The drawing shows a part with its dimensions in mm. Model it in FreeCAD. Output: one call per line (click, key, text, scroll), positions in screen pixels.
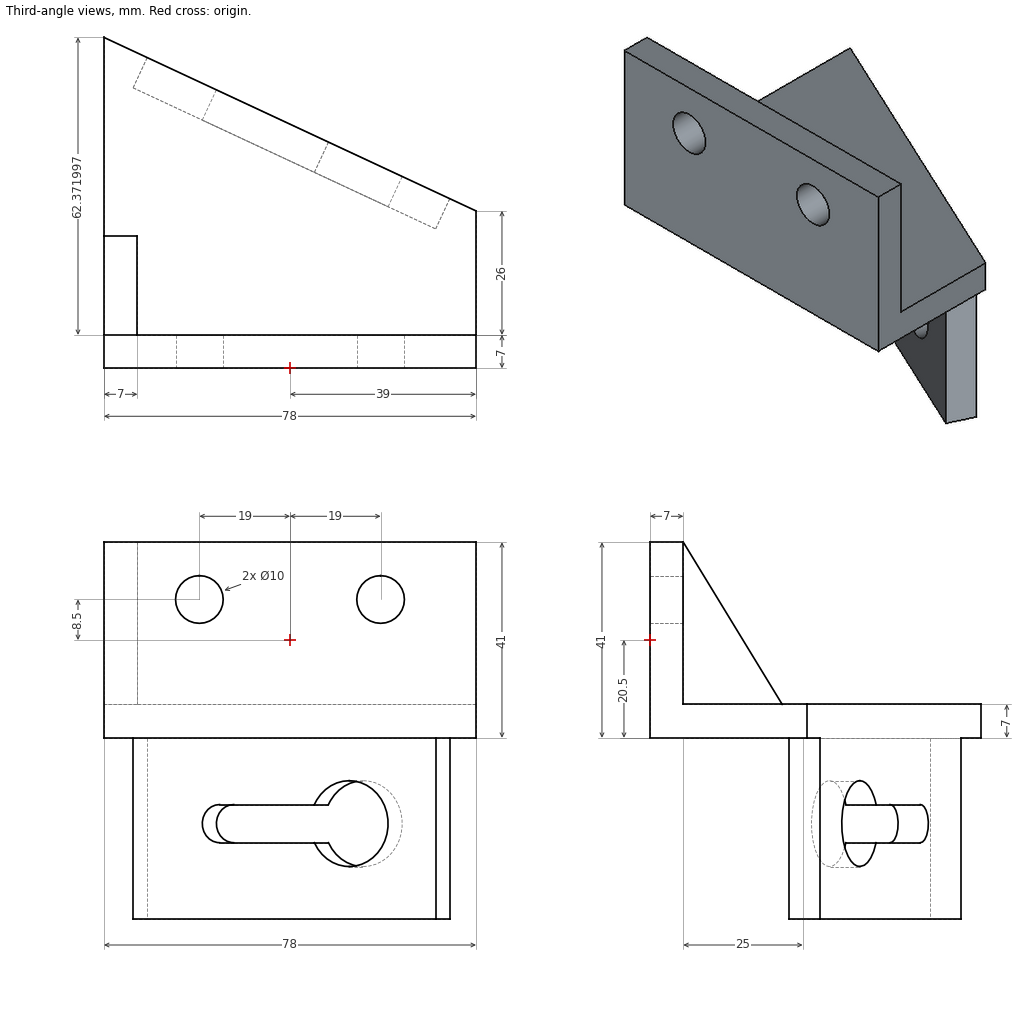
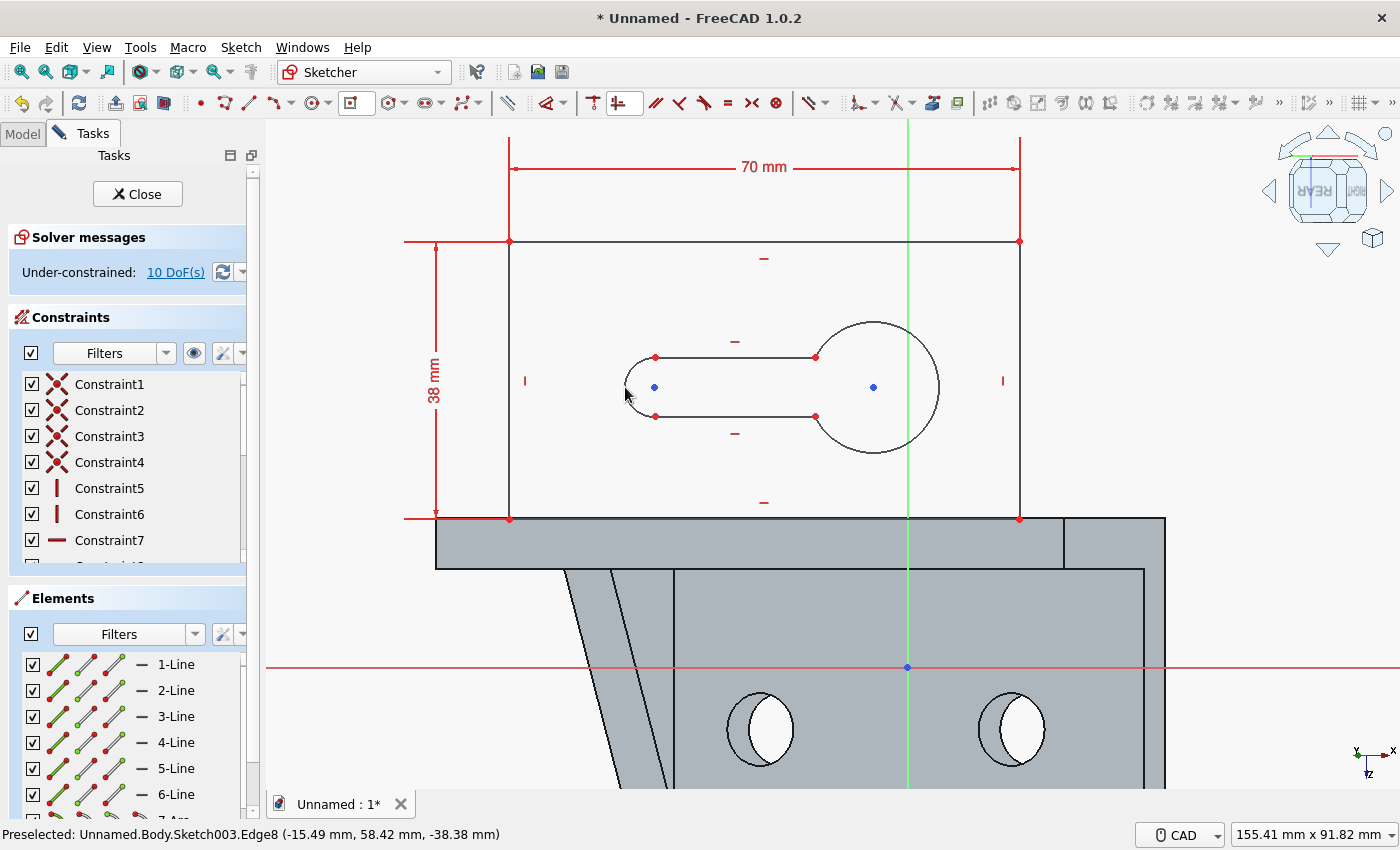
click(703, 358)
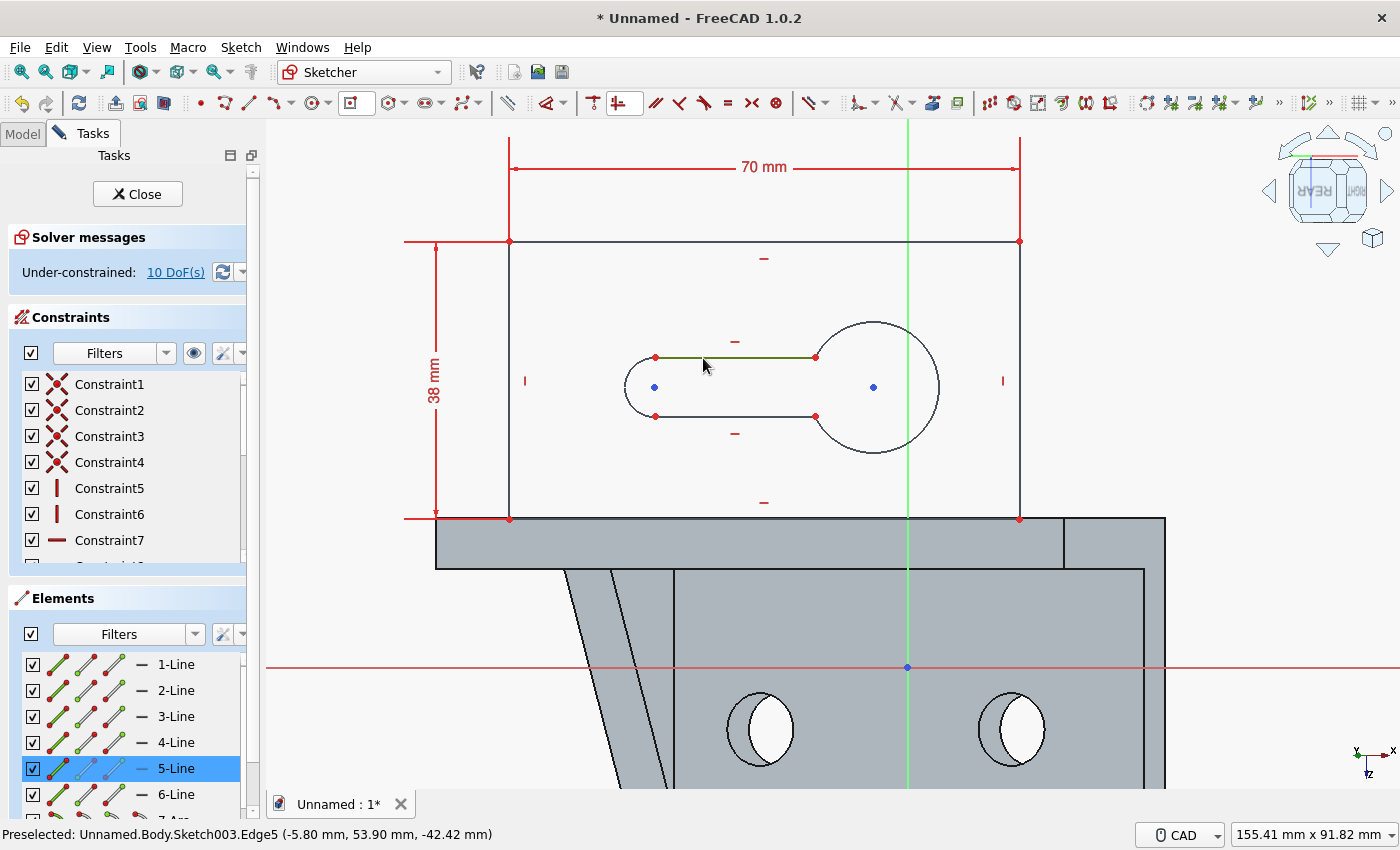
click(631, 370)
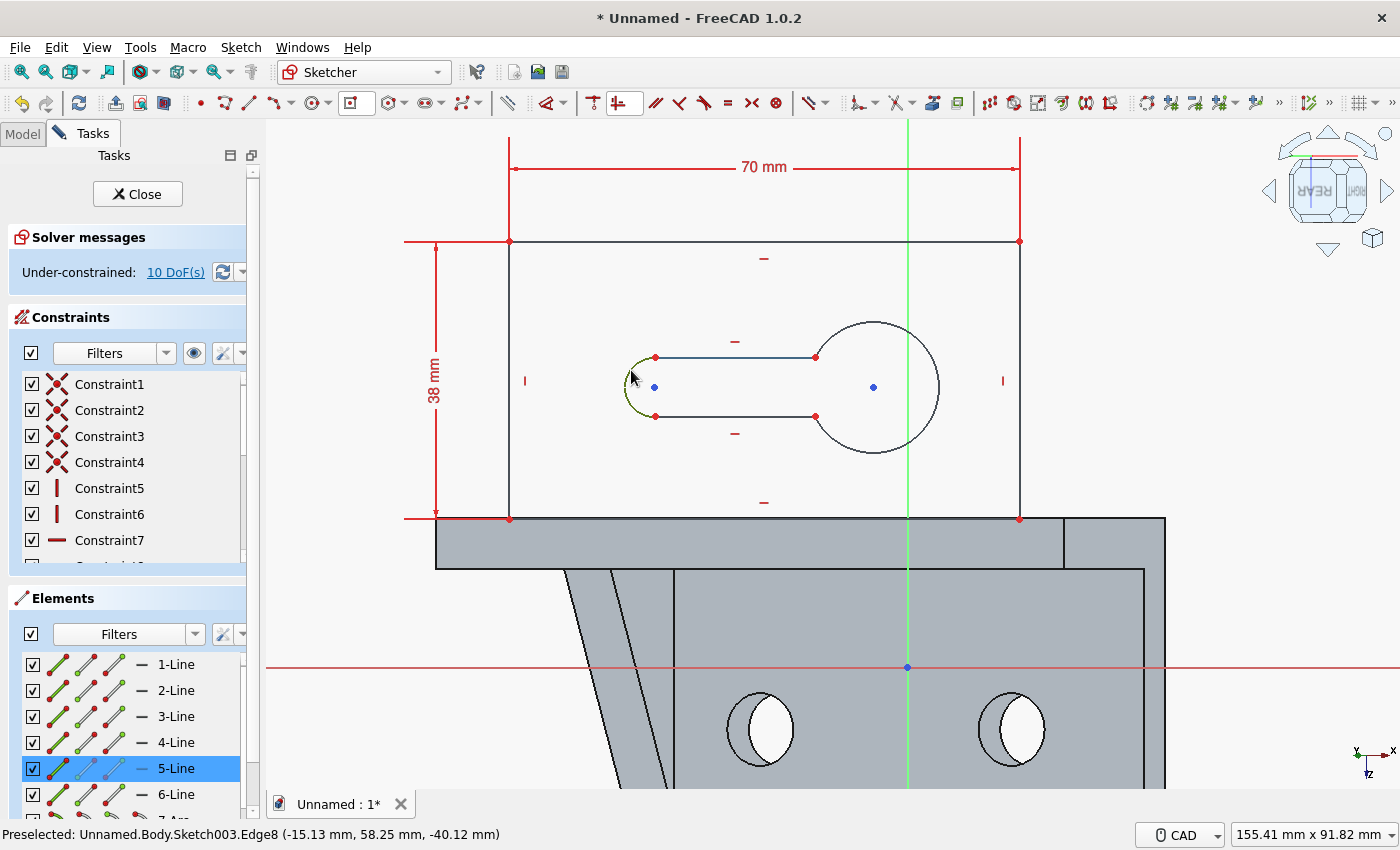
click(704, 104)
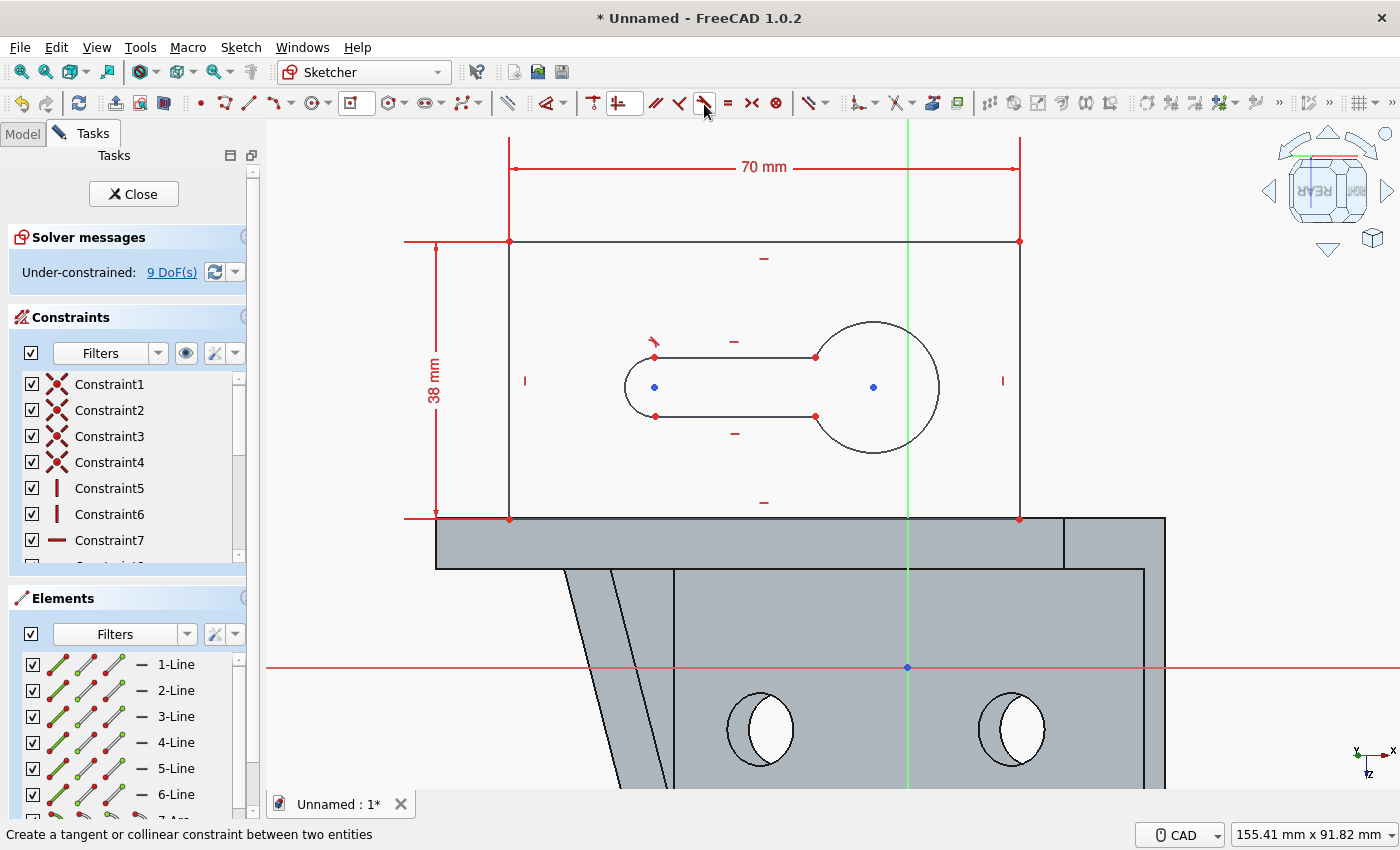
click(767, 417)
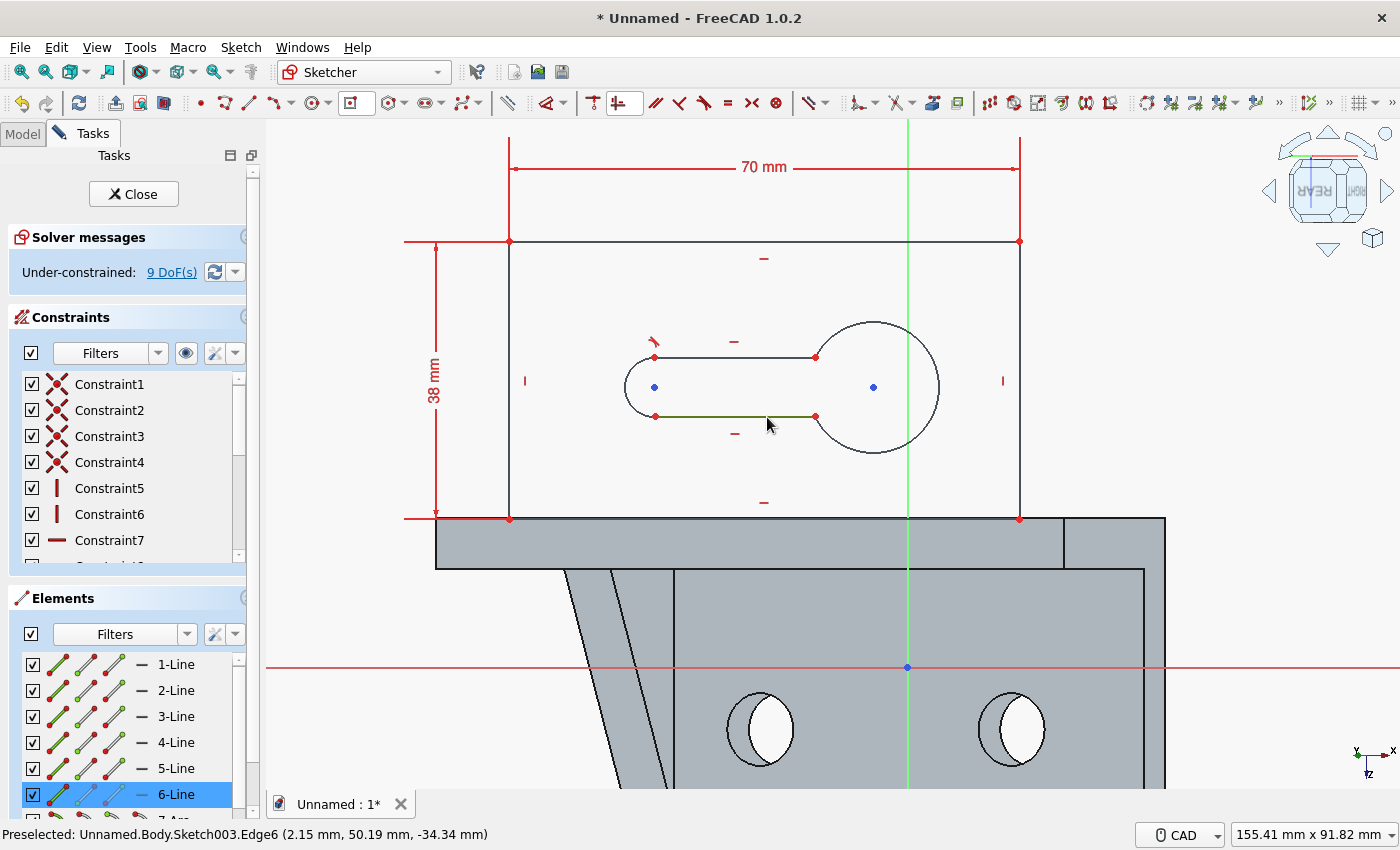
click(631, 370)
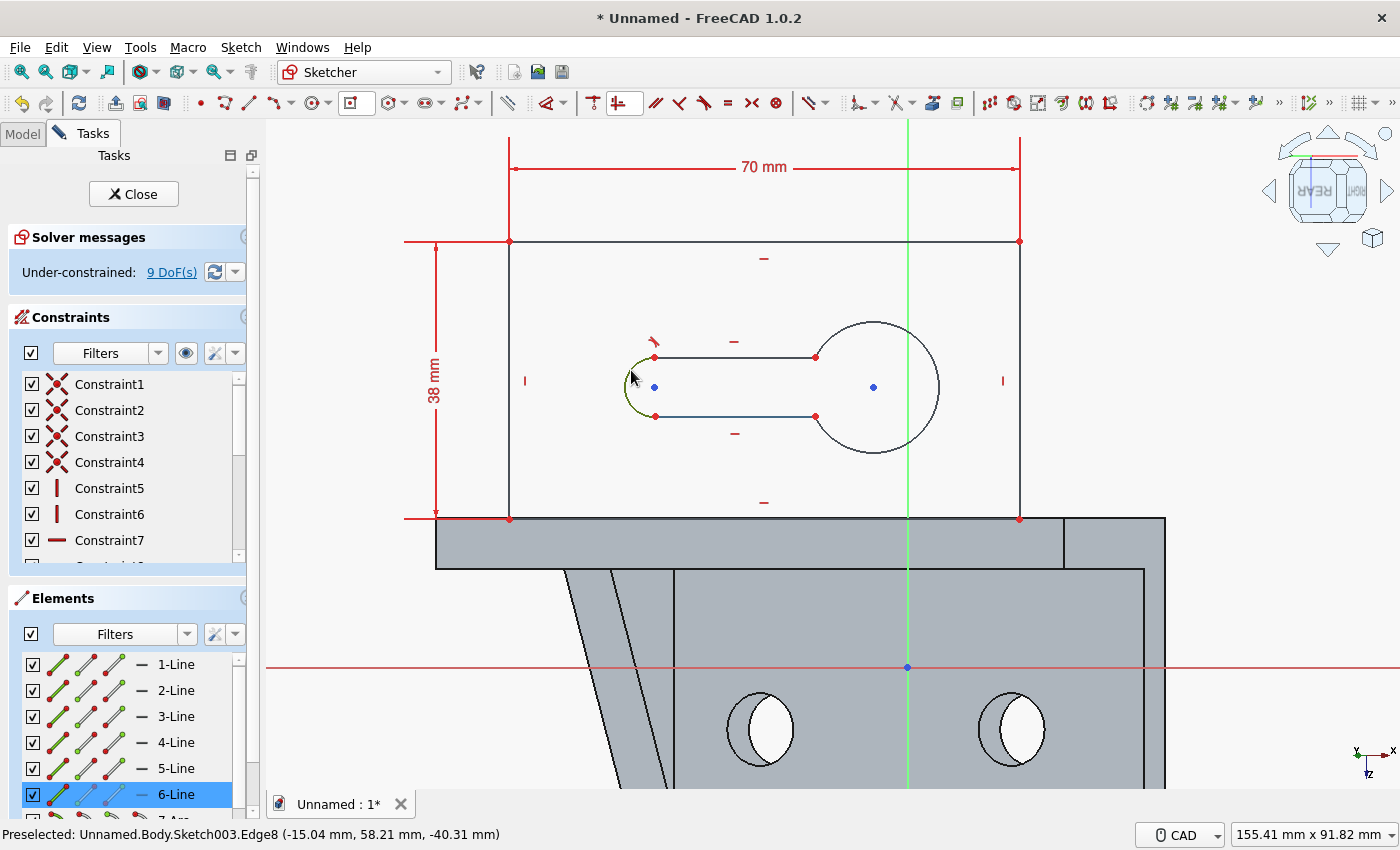
click(704, 104)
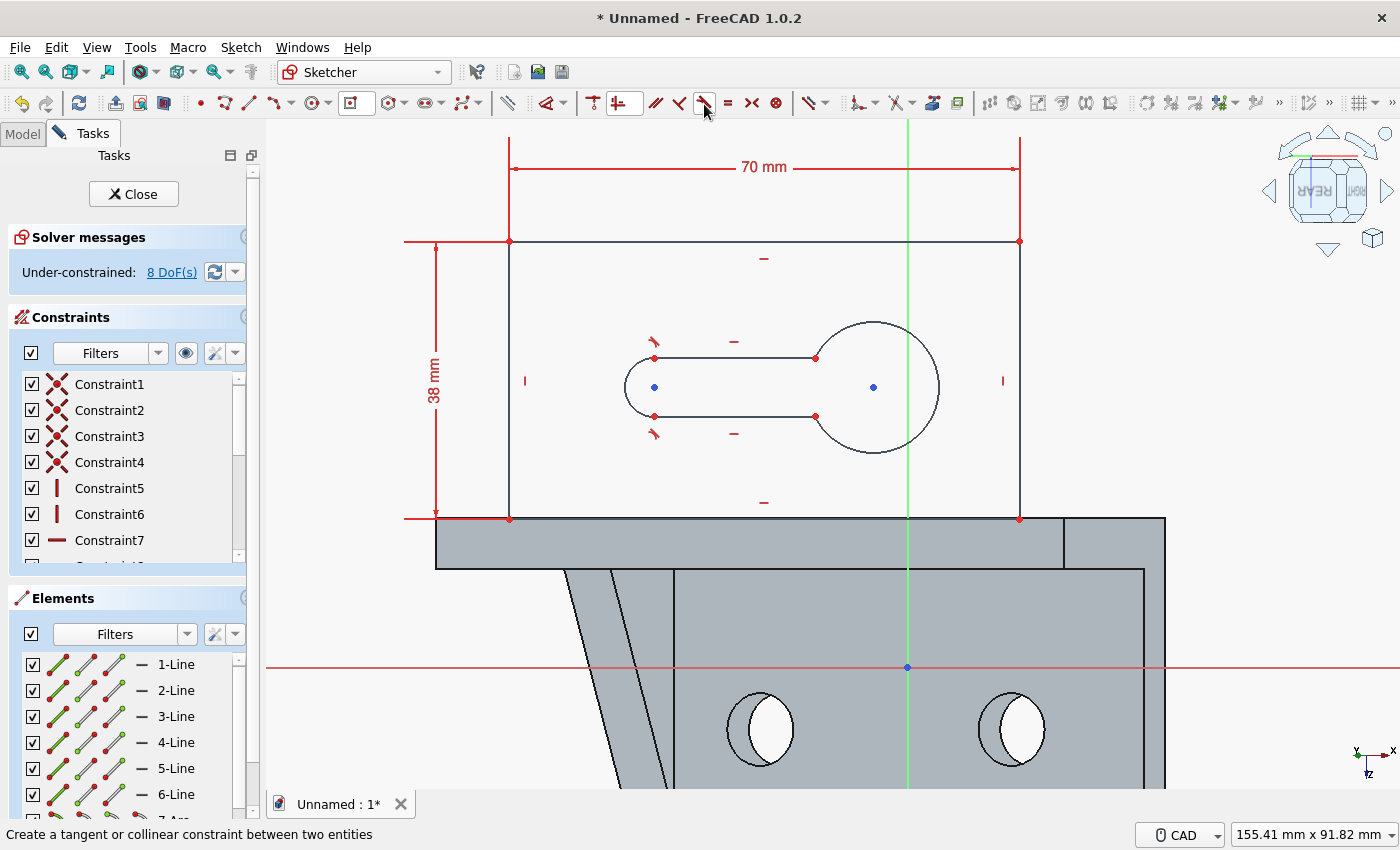
click(546, 104)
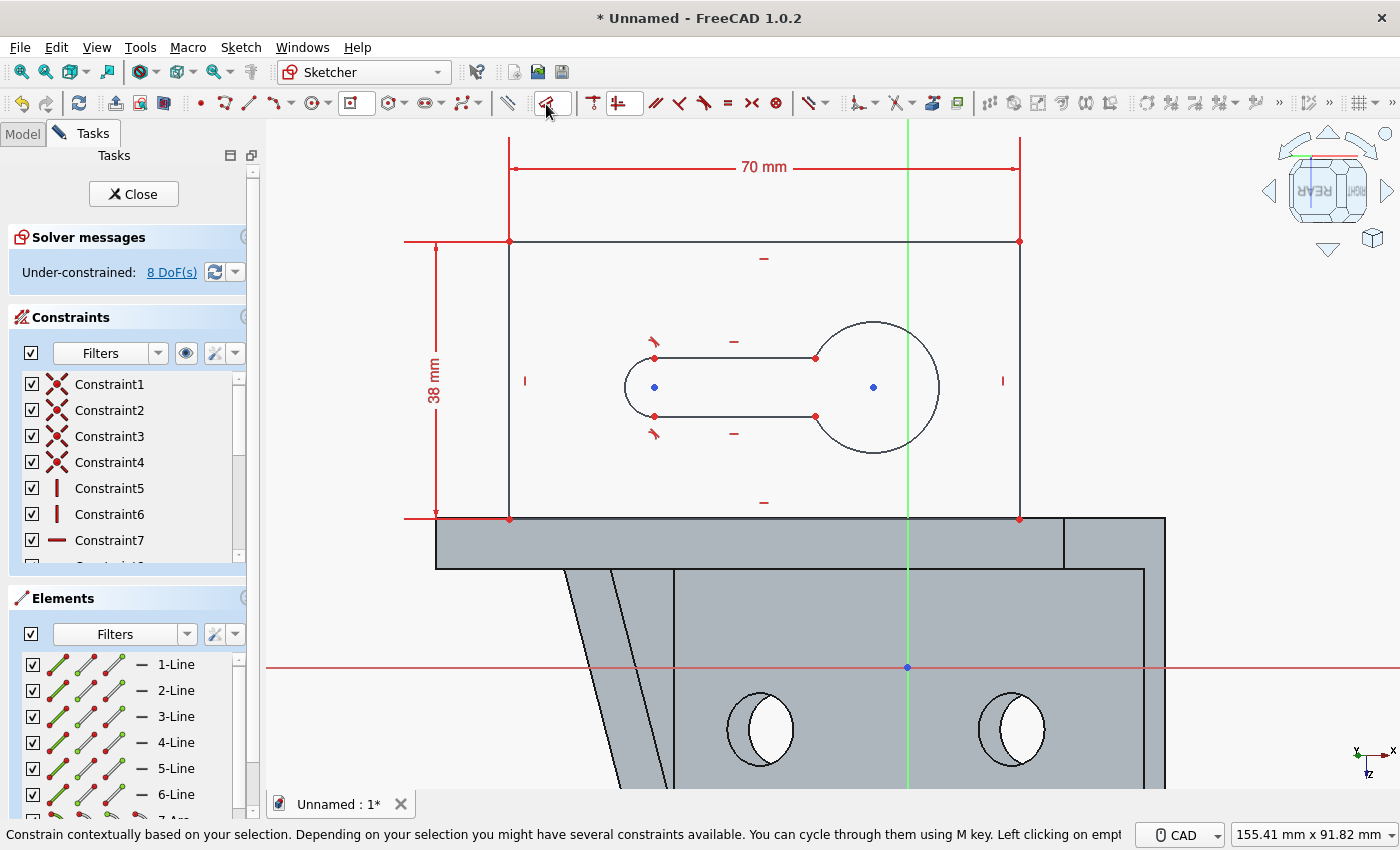
click(905, 445)
click(874, 485)